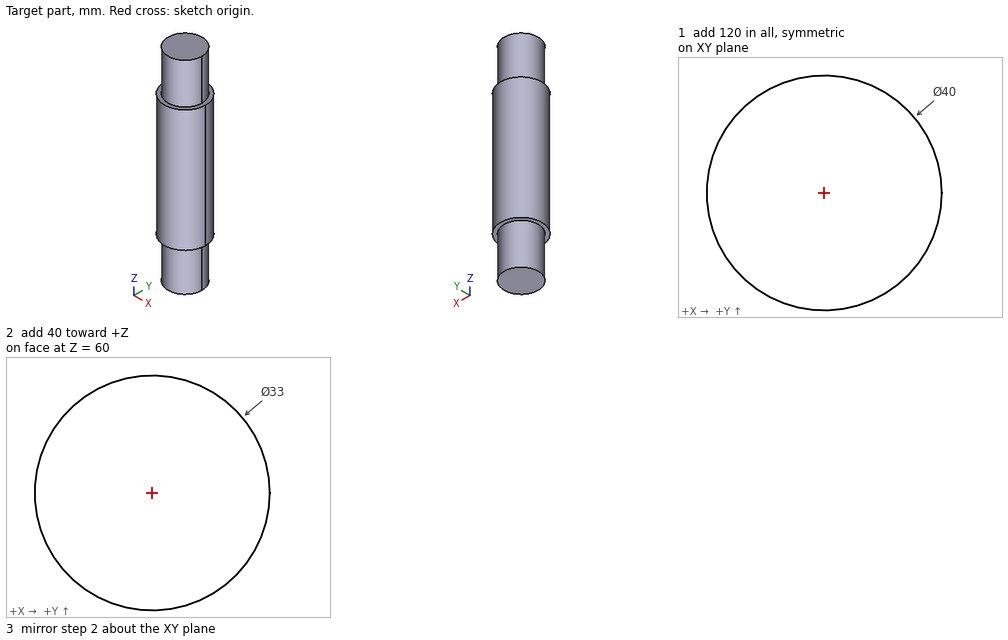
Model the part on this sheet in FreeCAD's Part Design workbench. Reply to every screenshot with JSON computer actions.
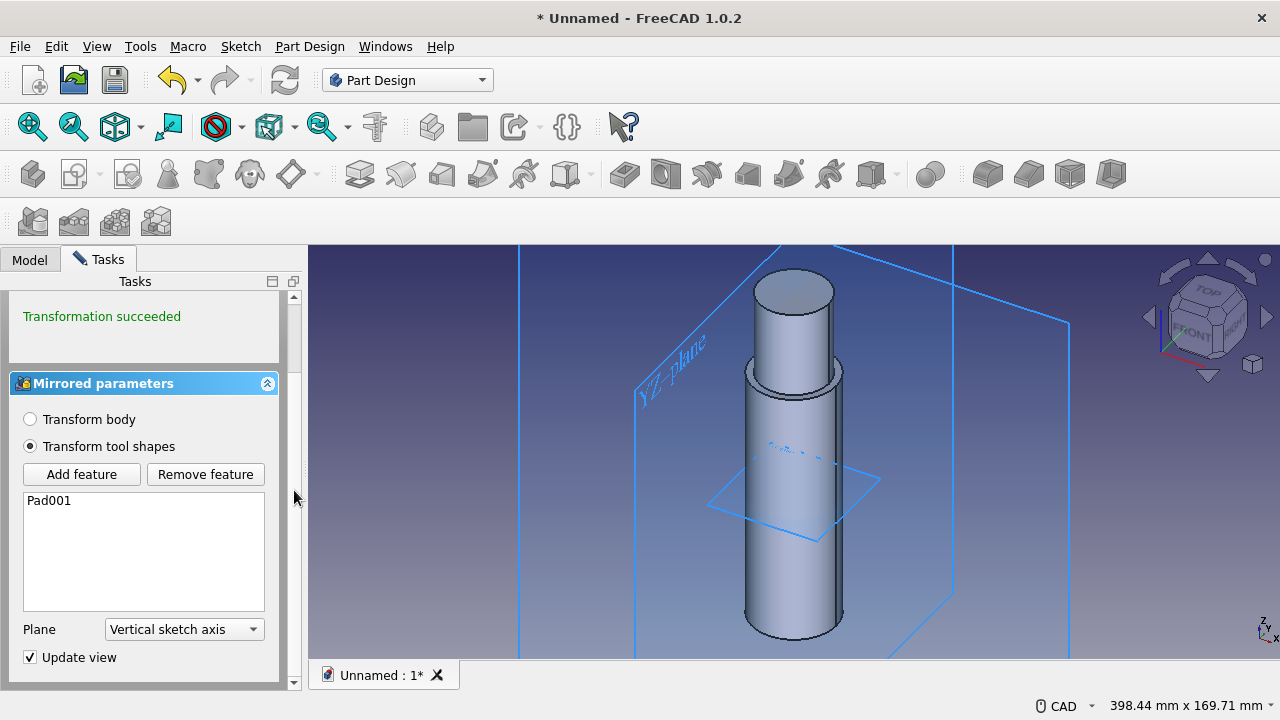
{"action": "left_click", "coordinate": [185, 630]}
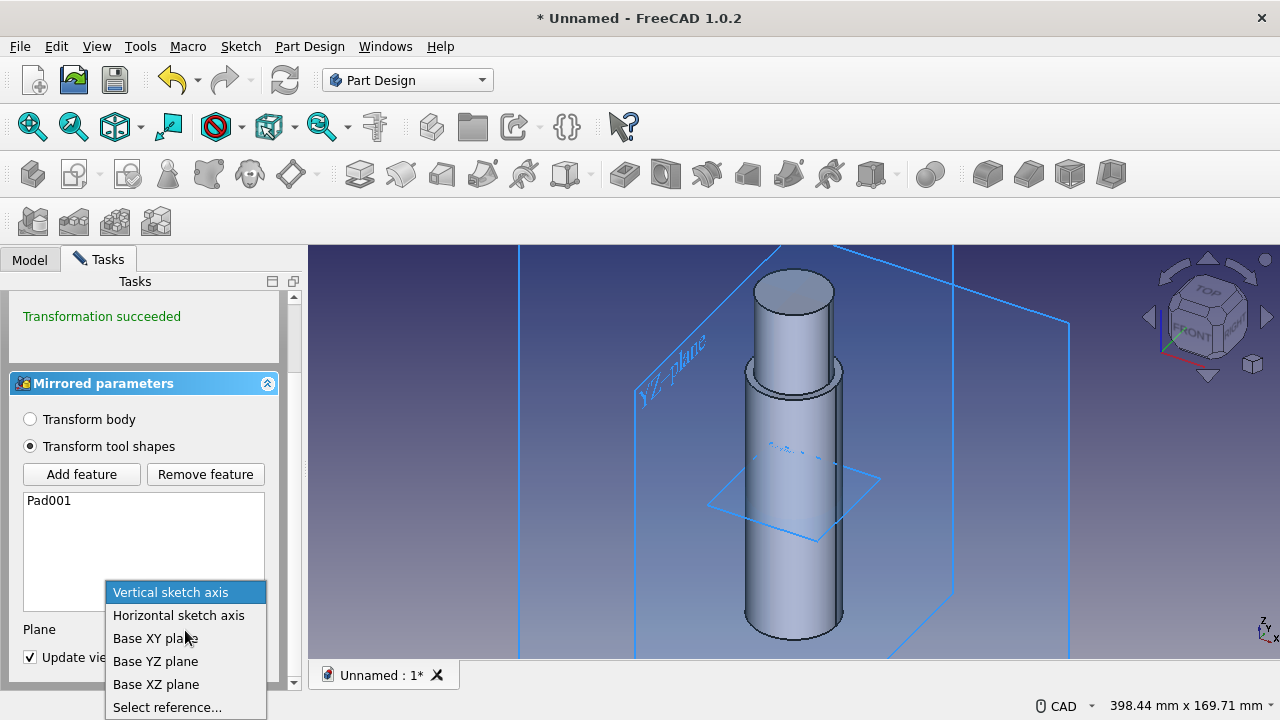
{"action": "left_click", "coordinate": [184, 638]}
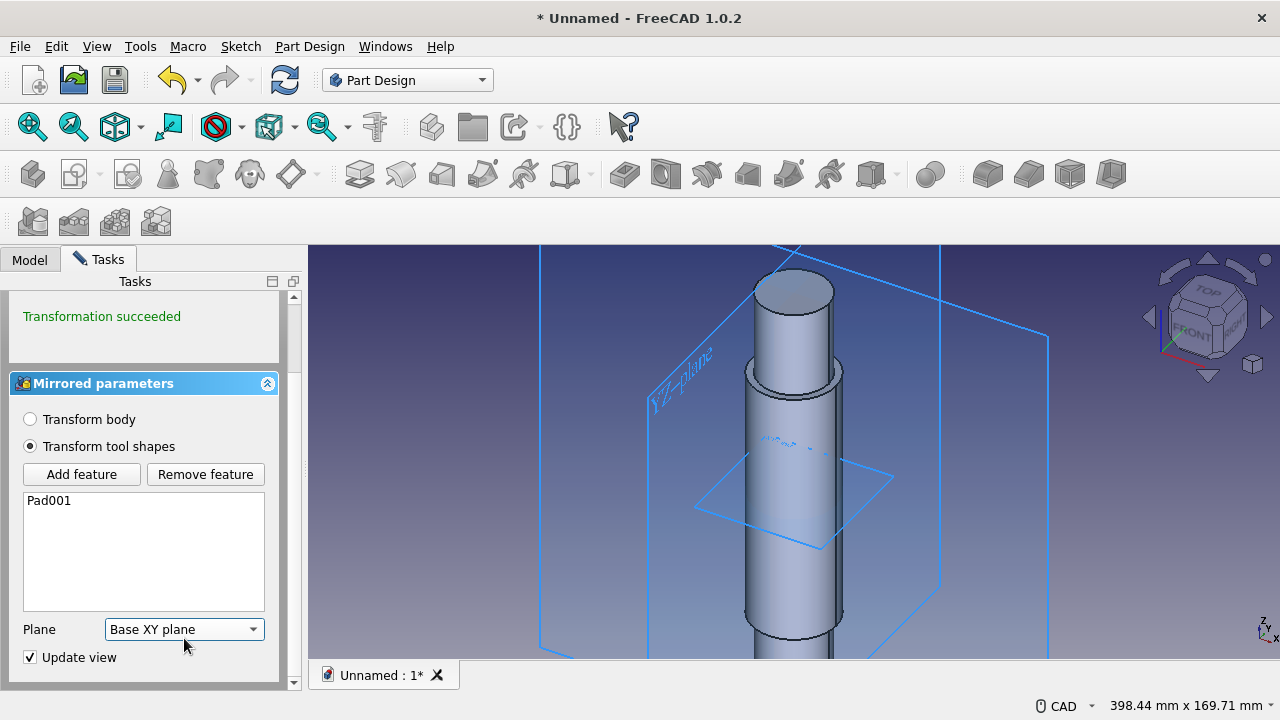
{"action": "scroll", "coordinate": [294, 490], "scroll_direction": "up", "scroll_amount": 3}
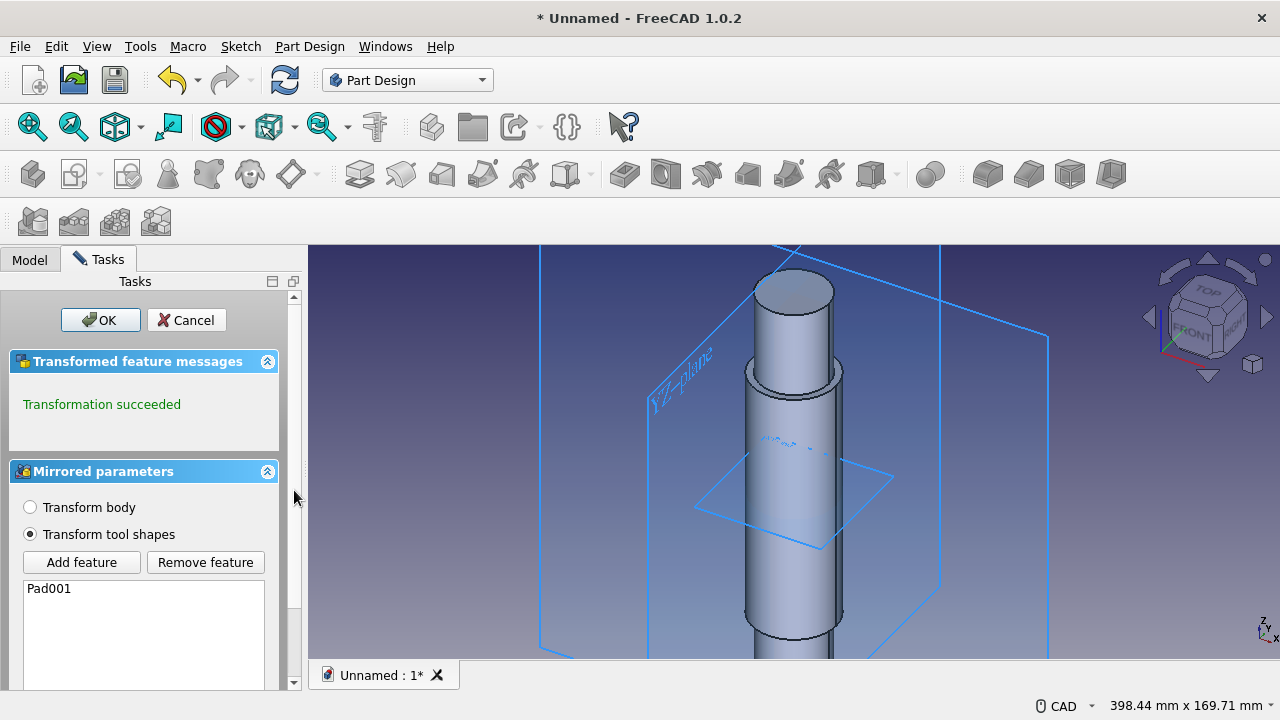
{"action": "left_click", "coordinate": [101, 320]}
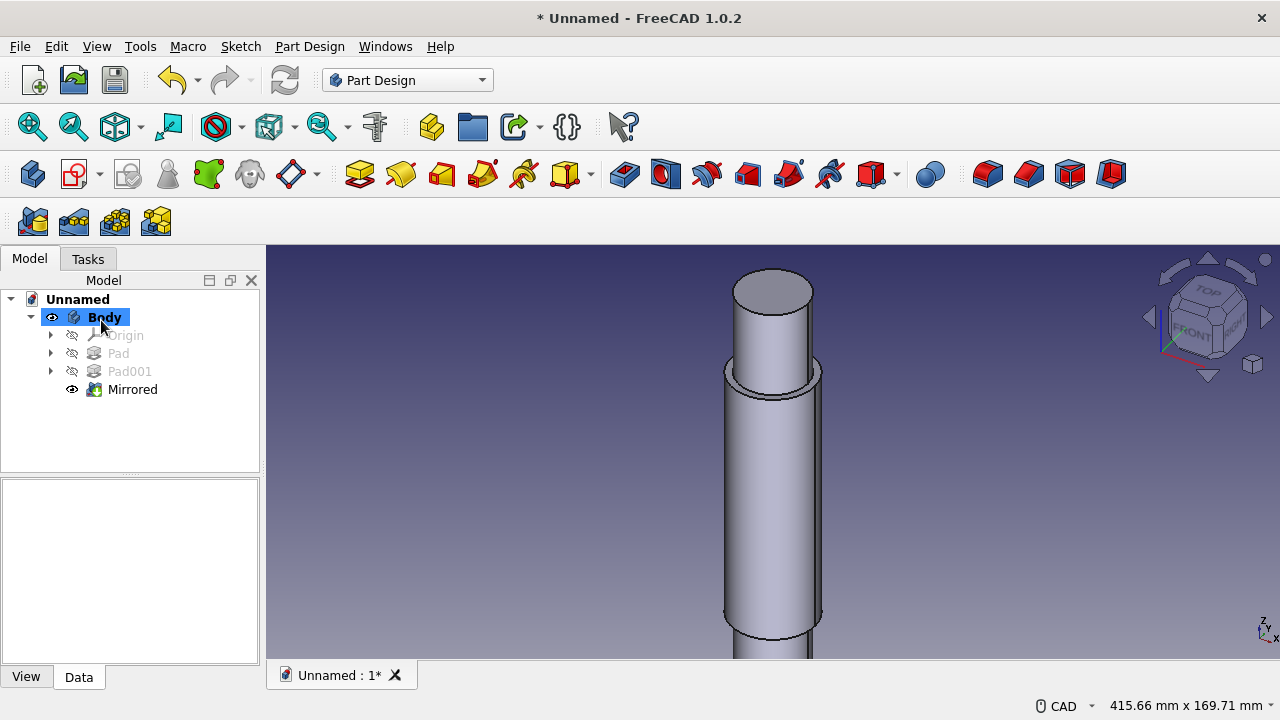
{"action": "key", "text": "0"}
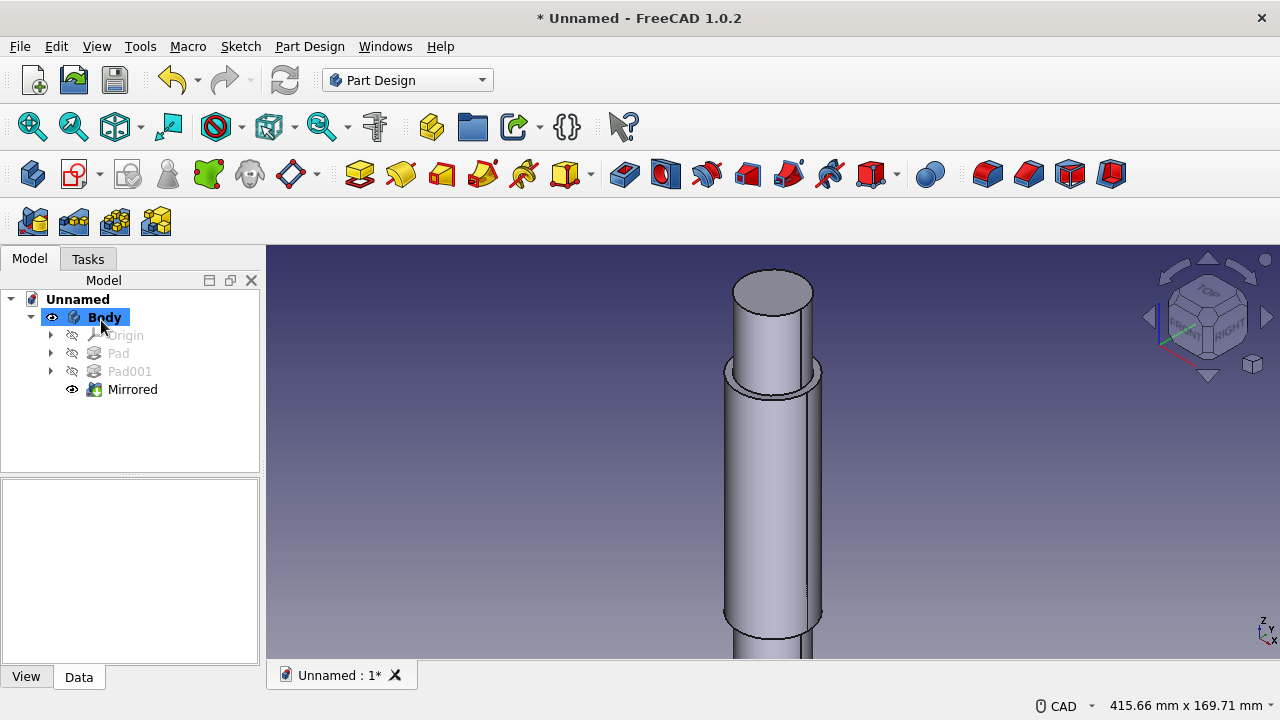
{"action": "left_click", "coordinate": [33, 128]}